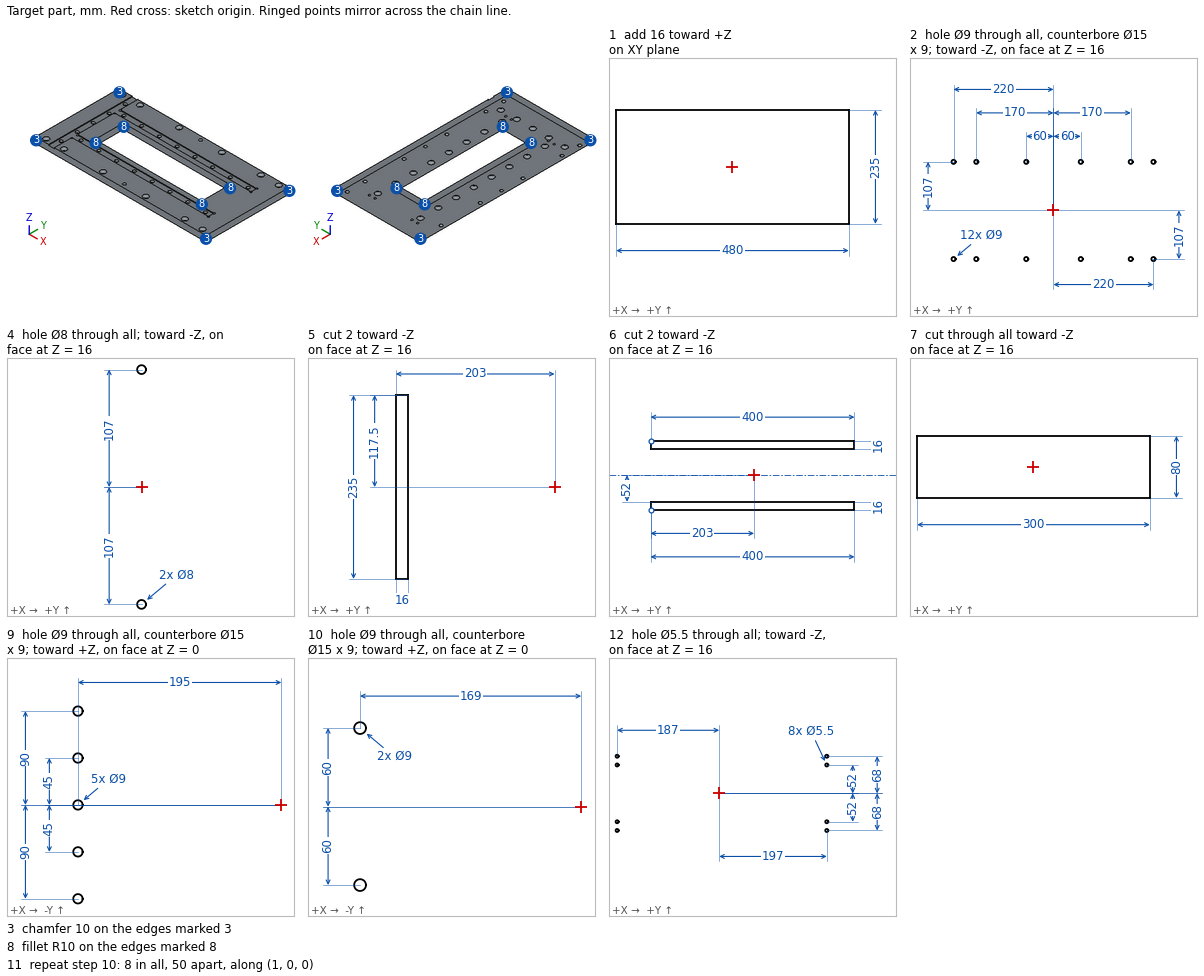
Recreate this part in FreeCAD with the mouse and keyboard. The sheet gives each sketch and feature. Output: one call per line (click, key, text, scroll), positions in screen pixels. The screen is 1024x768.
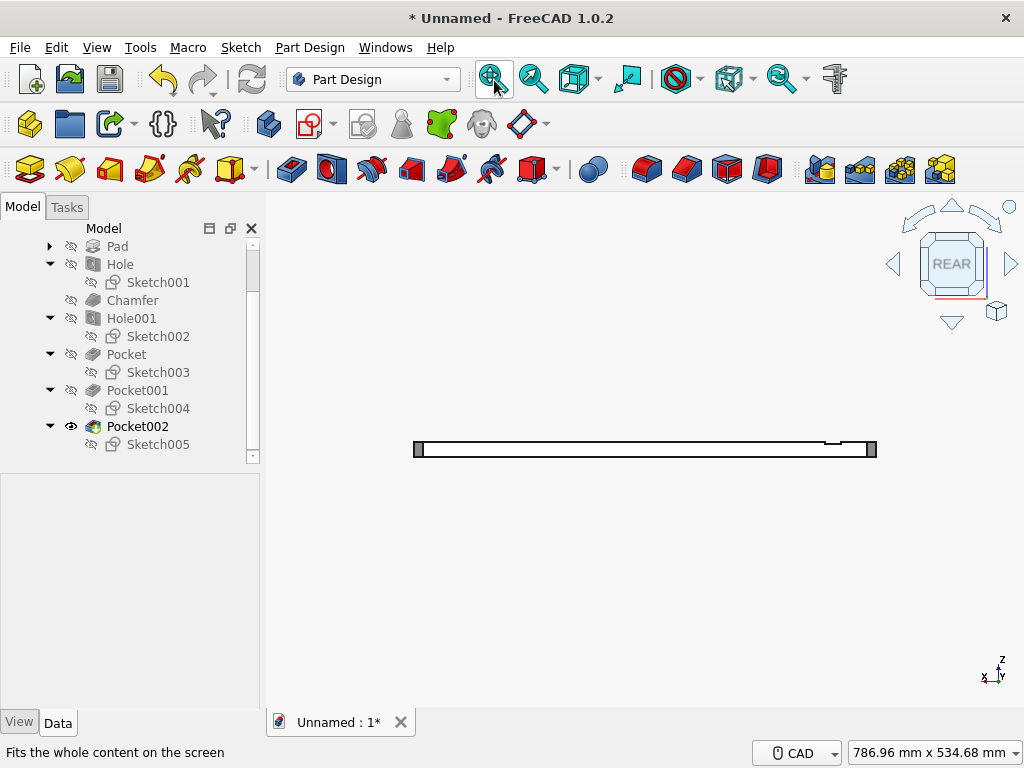
scroll(501, 449, up, 5)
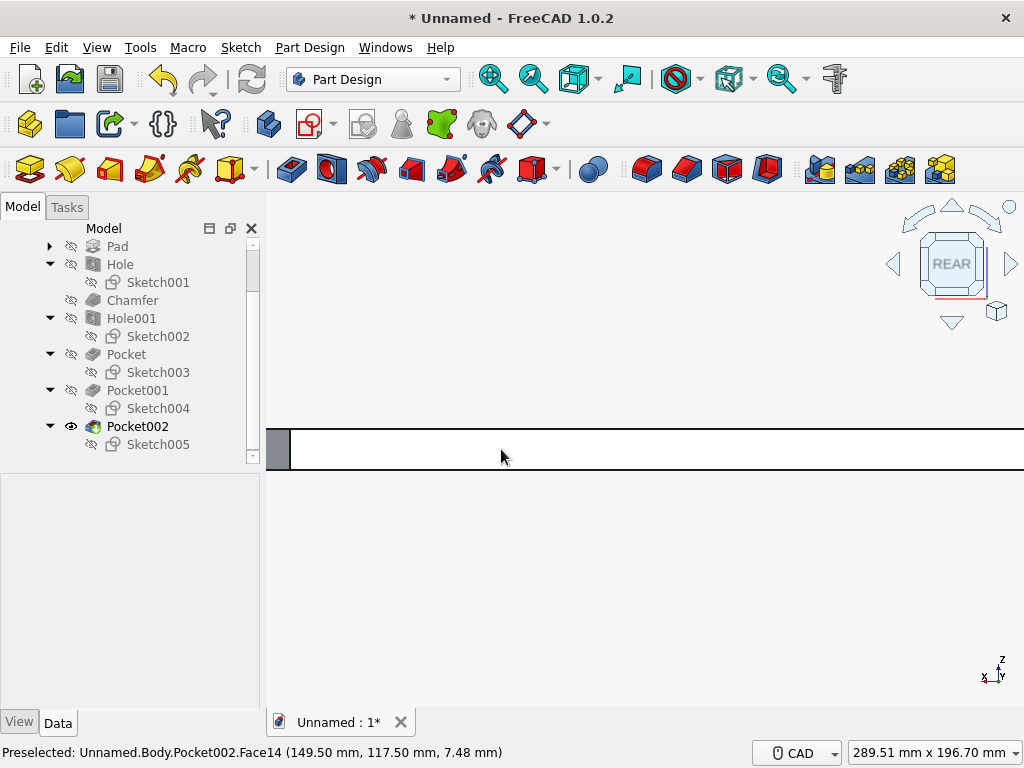
click(494, 80)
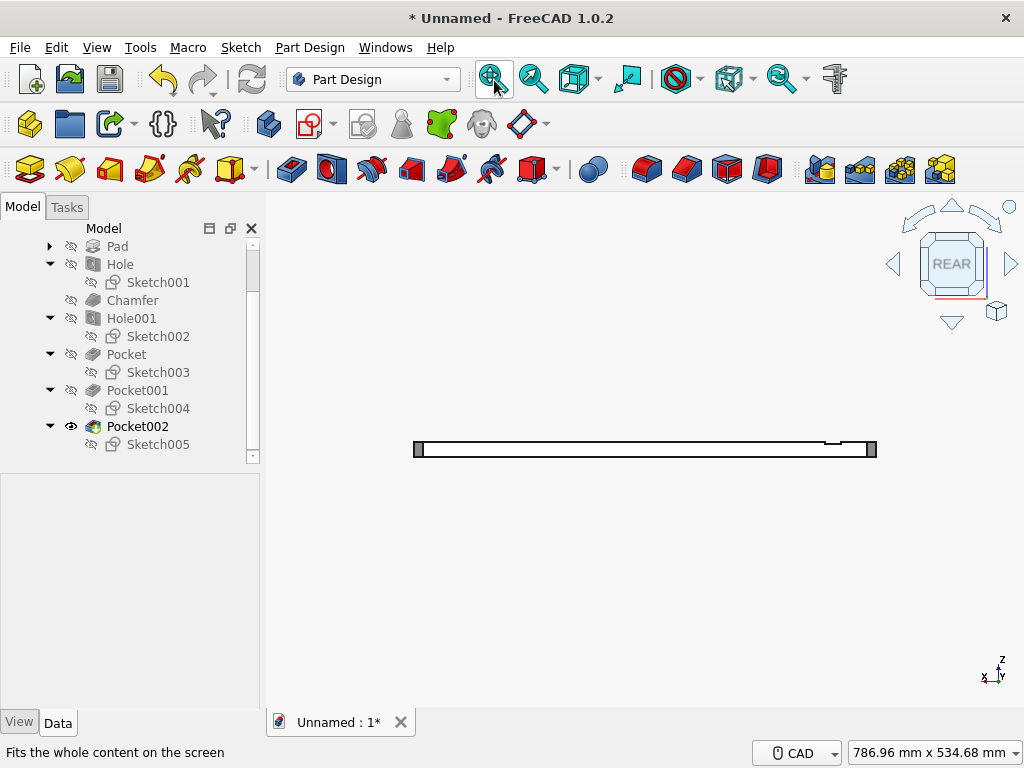
key(6)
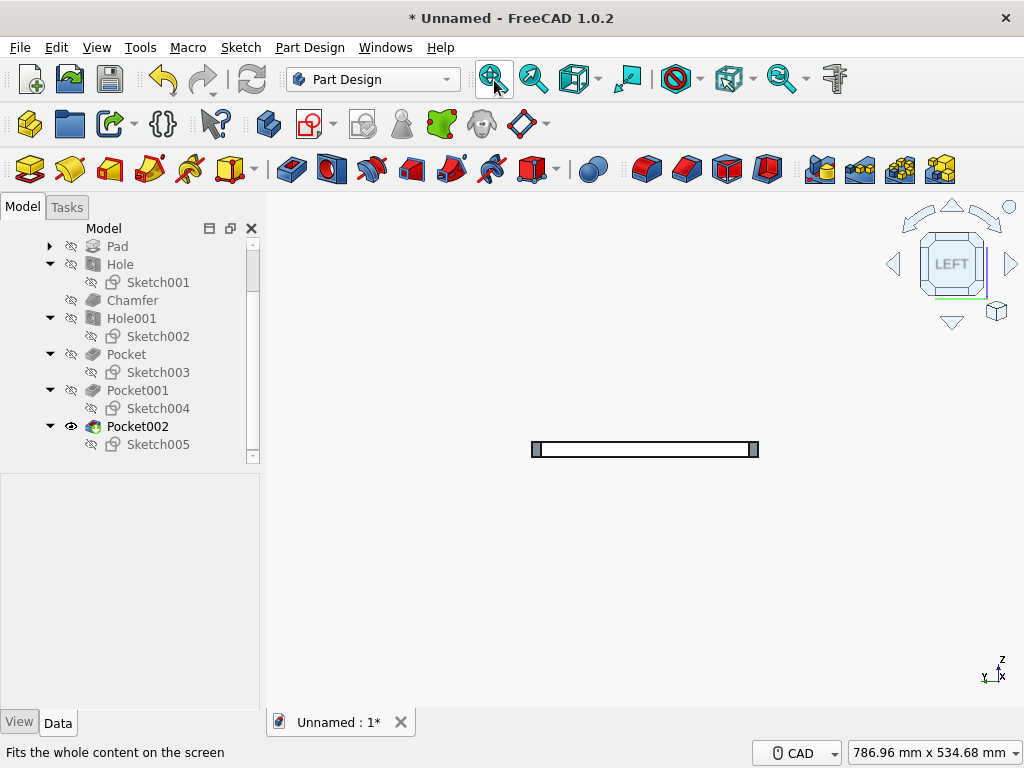
click(494, 80)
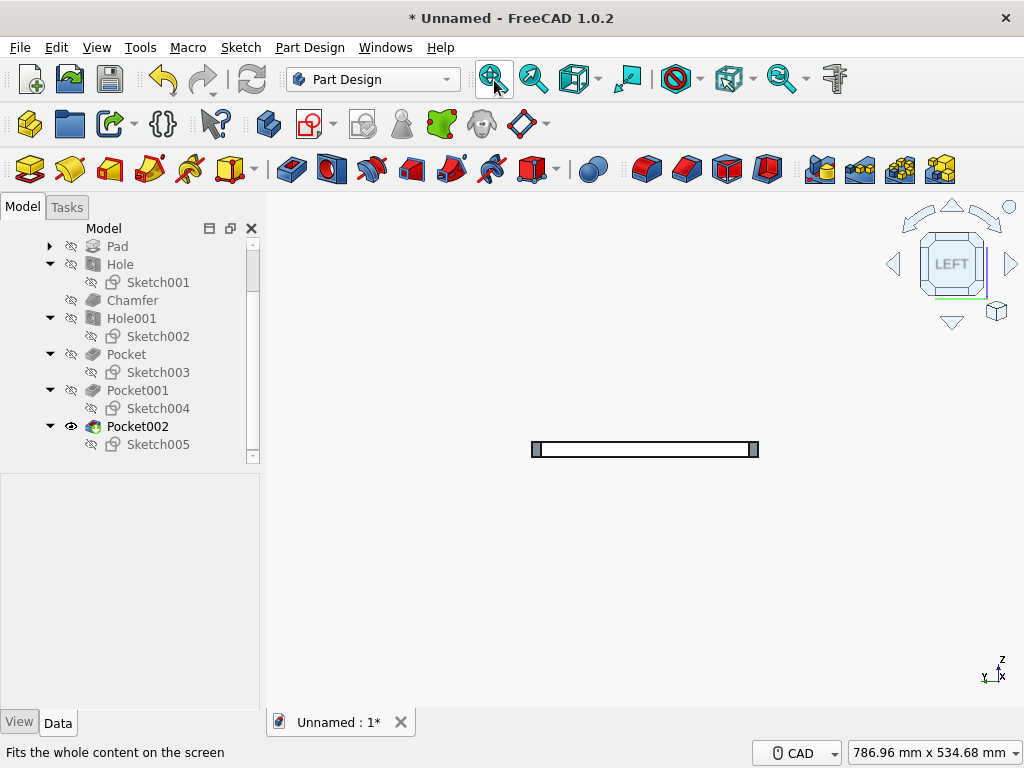
scroll(606, 448, up, 5)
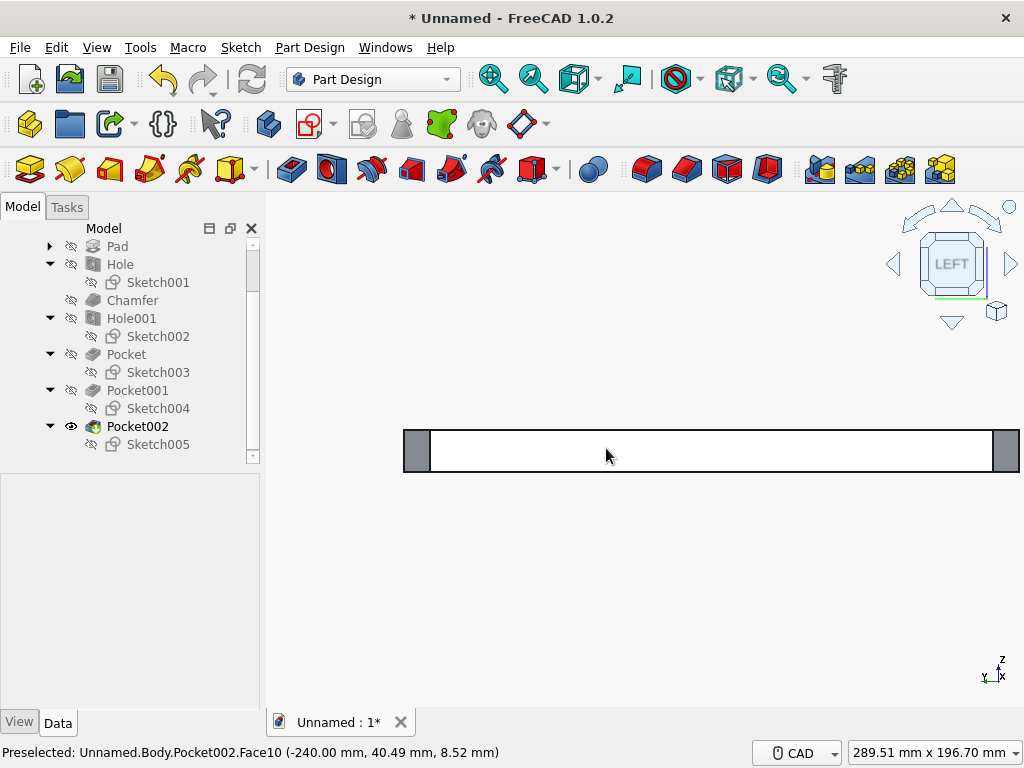
click(494, 80)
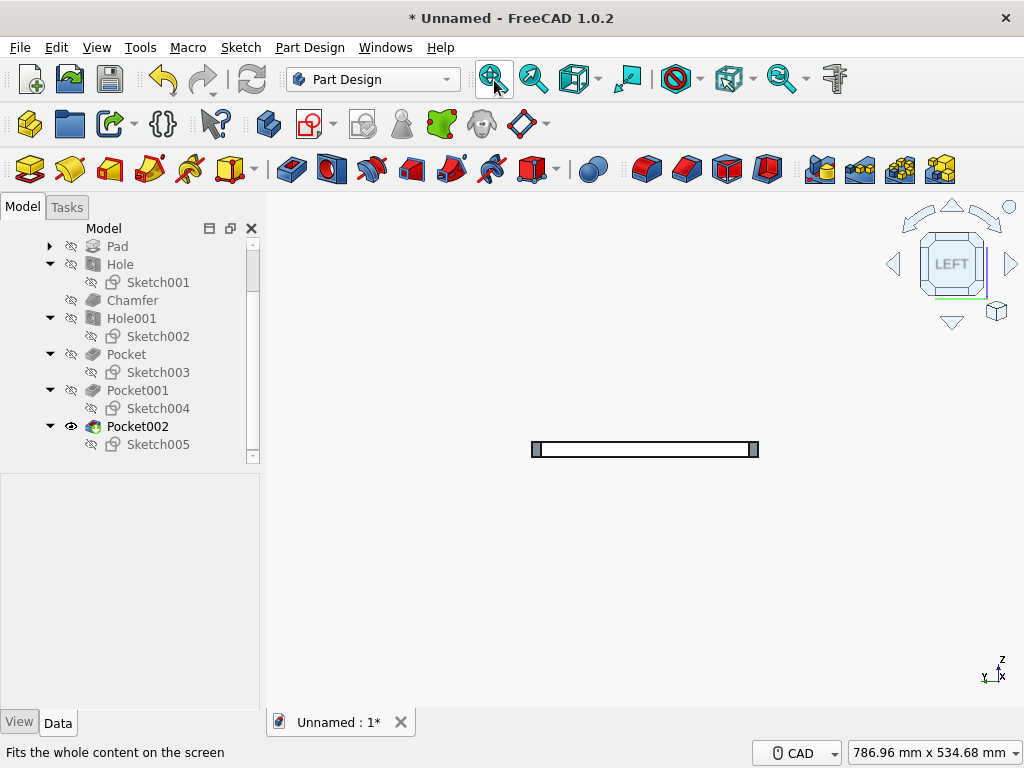
key(v)
key(3)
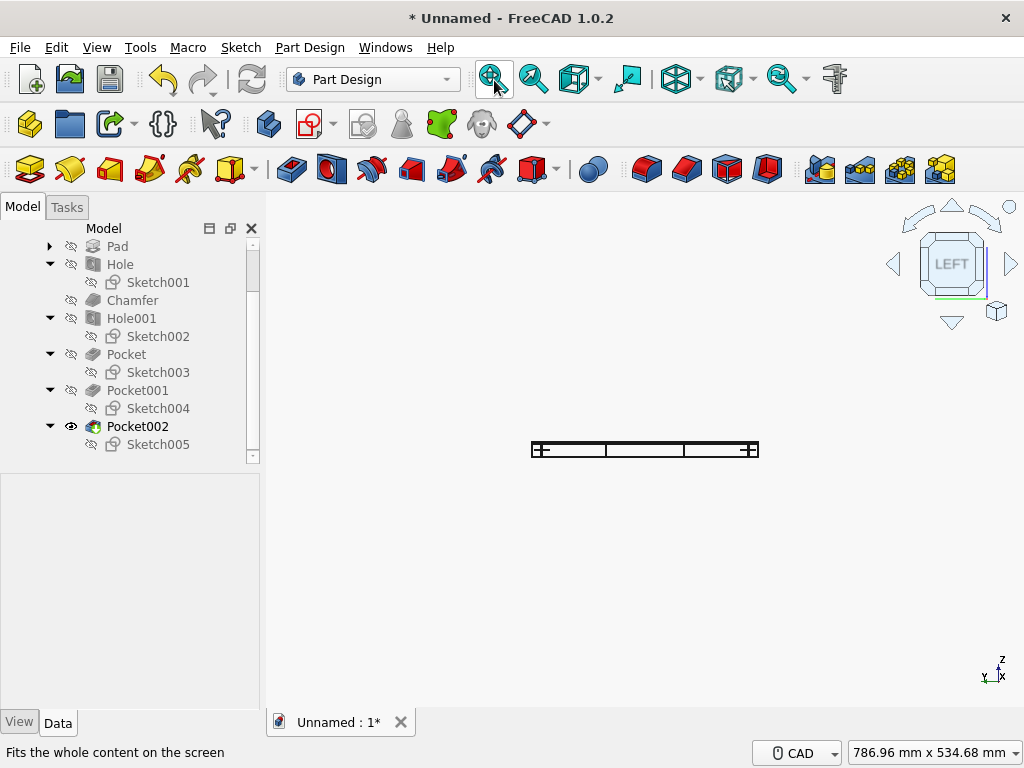
key(0)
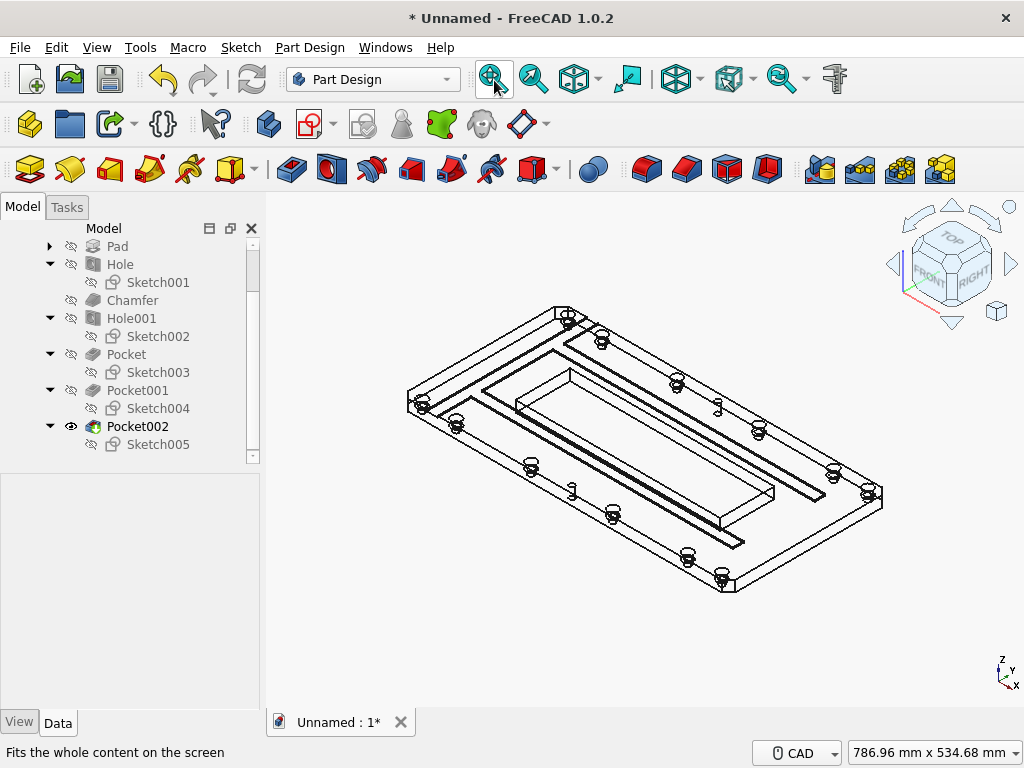
click(774, 494)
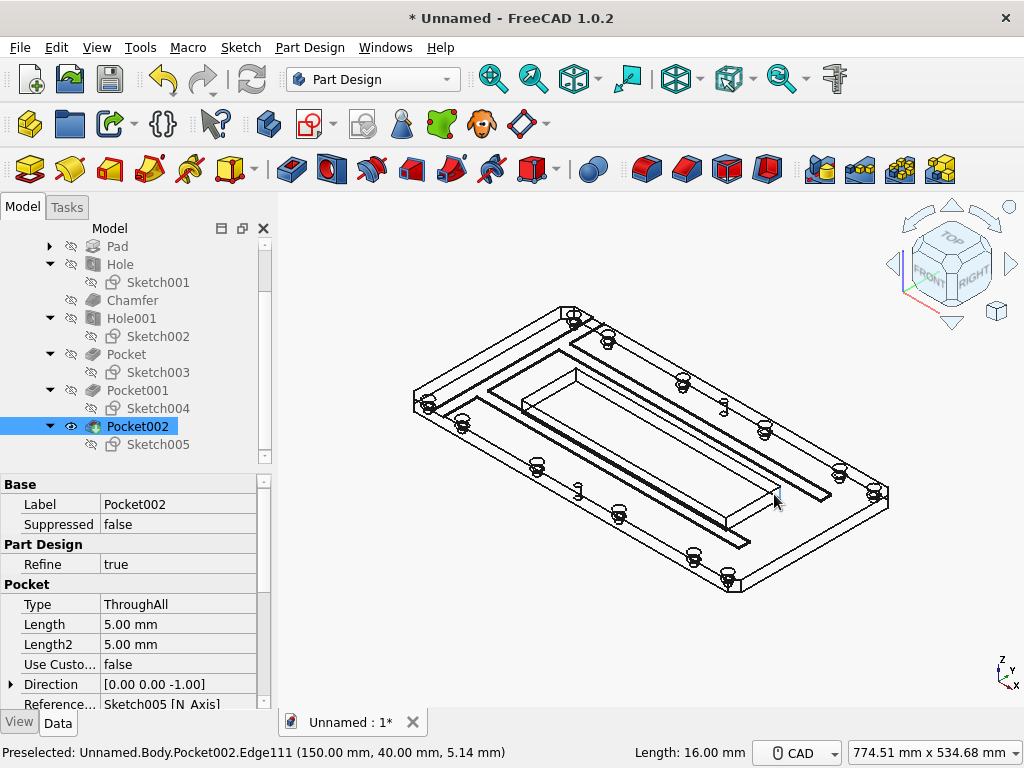
click(576, 375, ctrl)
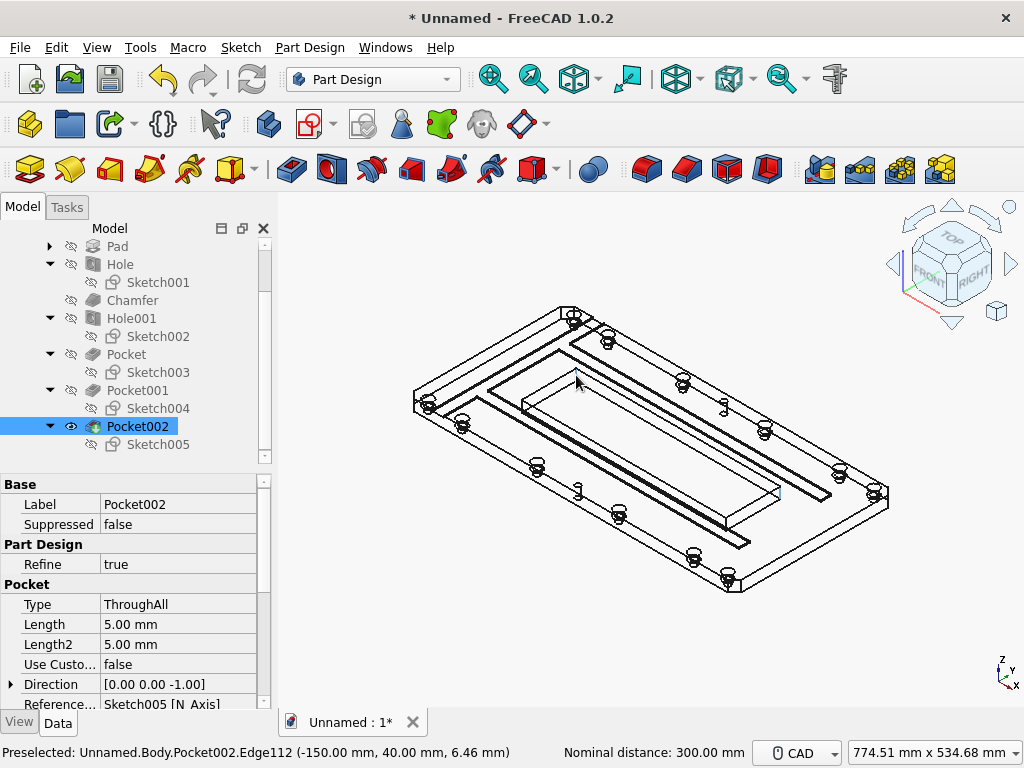
scroll(726, 523, up, 6)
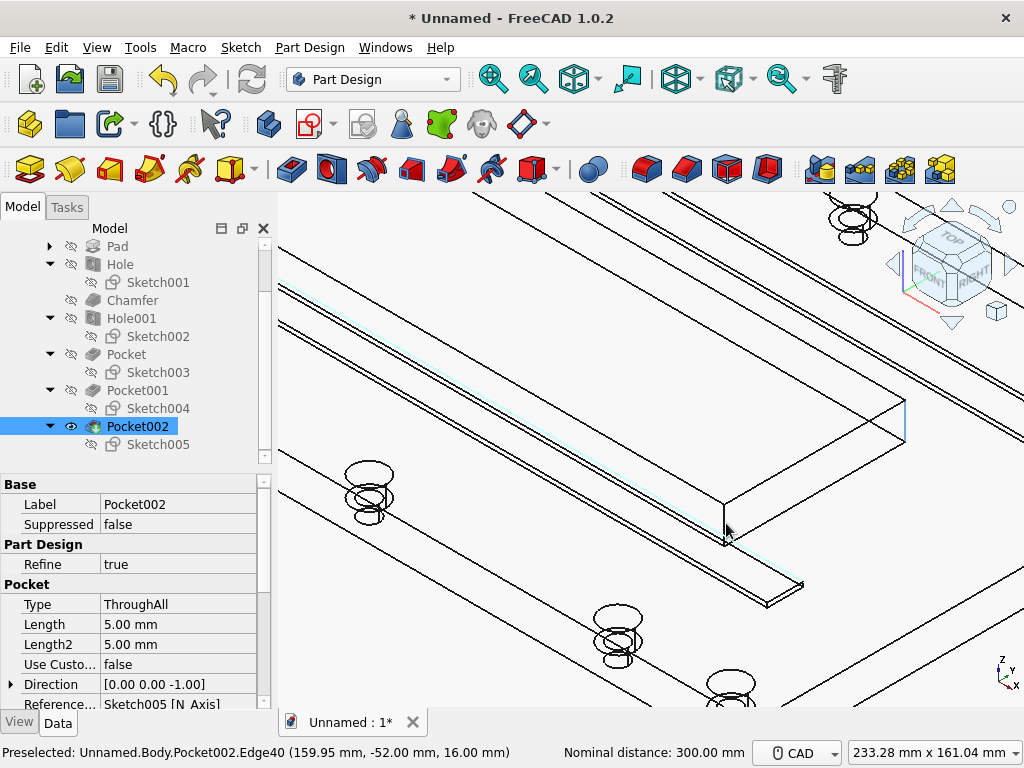
click(724, 525, ctrl)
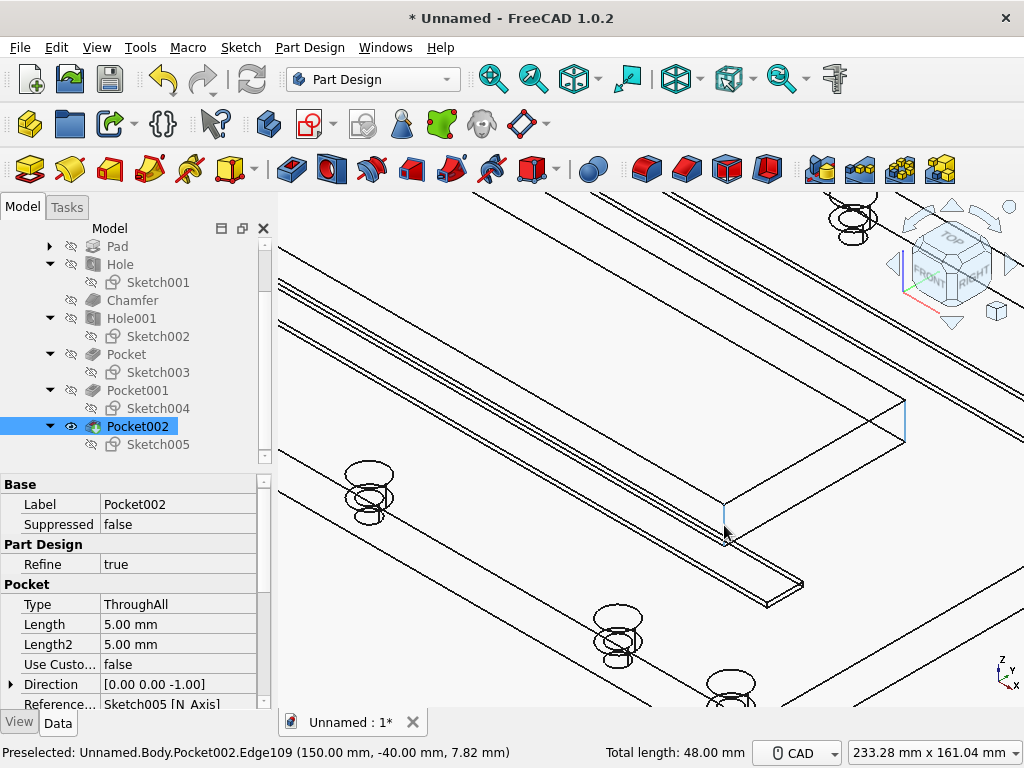
click(494, 80)